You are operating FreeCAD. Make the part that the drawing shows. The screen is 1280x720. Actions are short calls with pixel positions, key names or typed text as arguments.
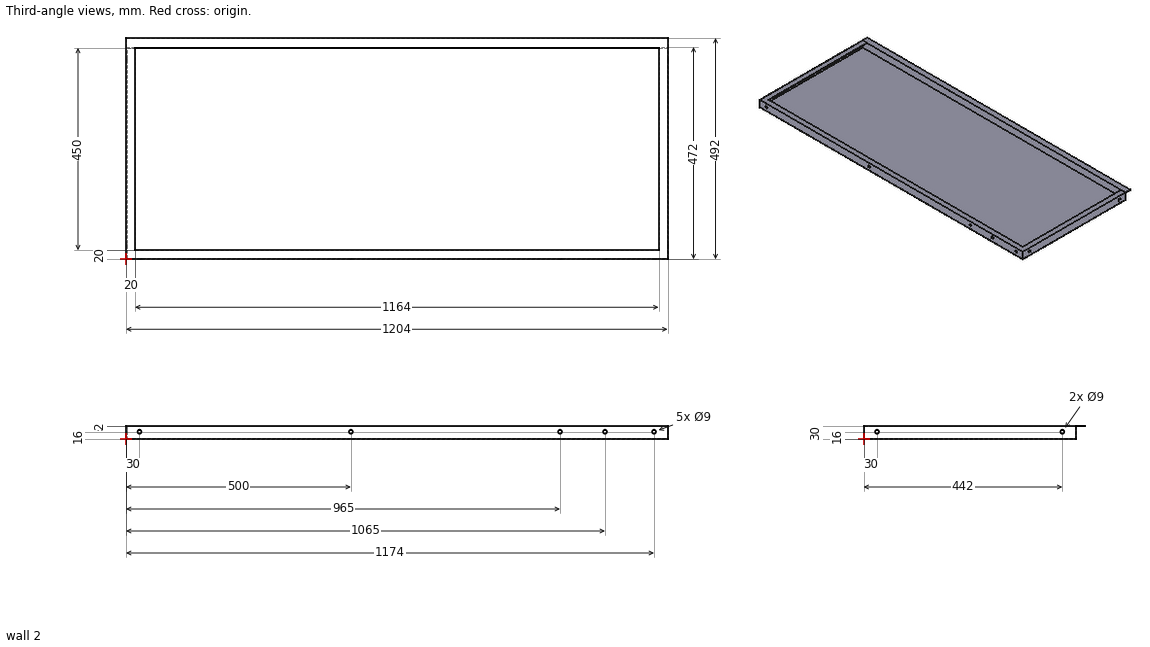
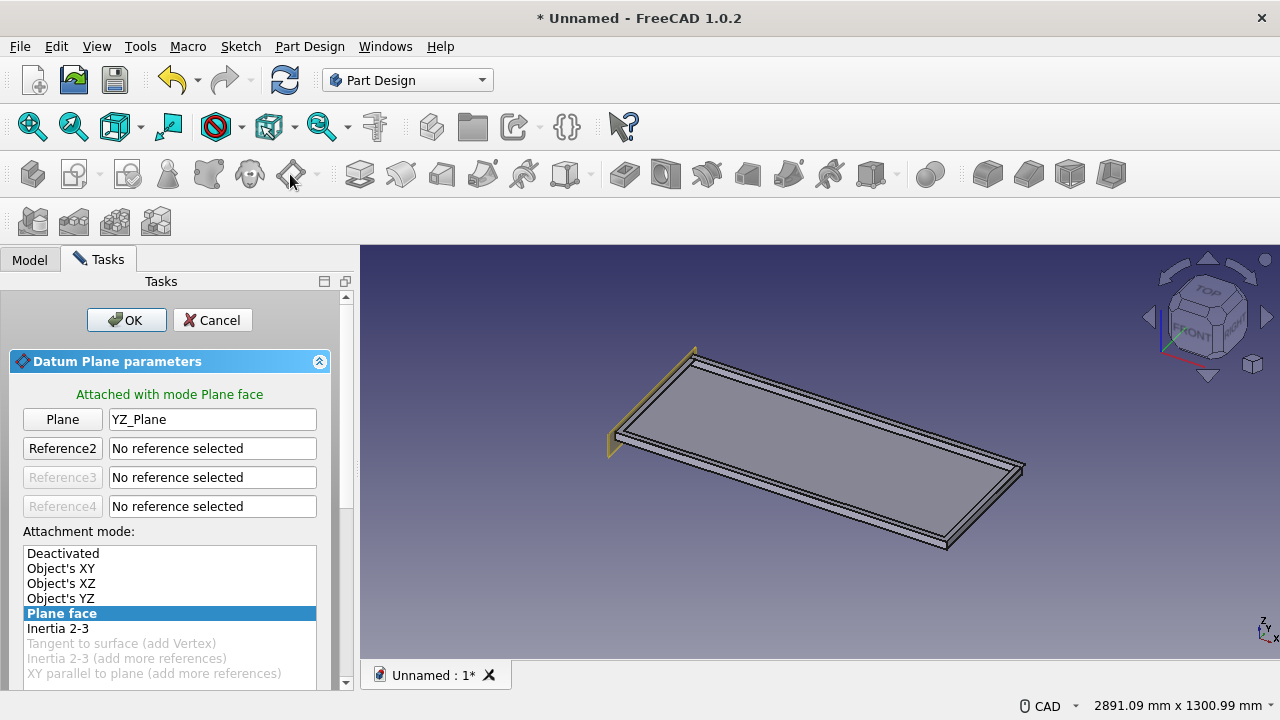
scroll(346, 490, down, 4)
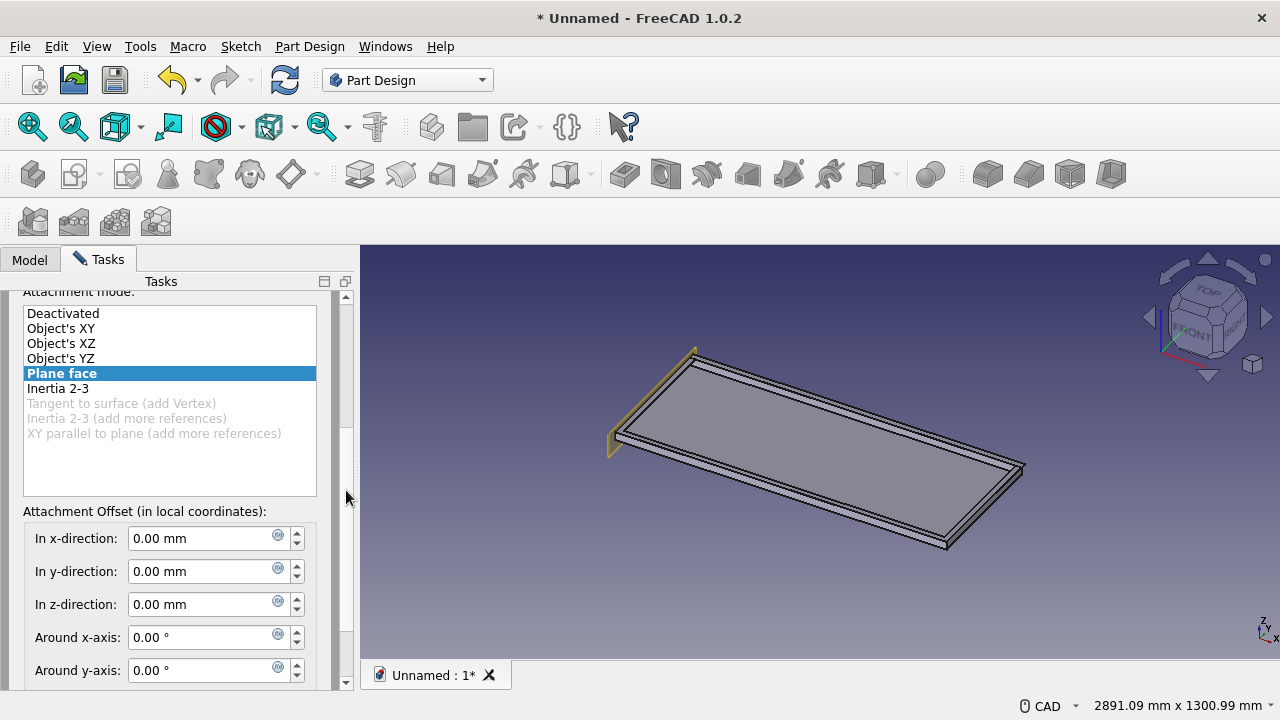
triple_click(210, 604)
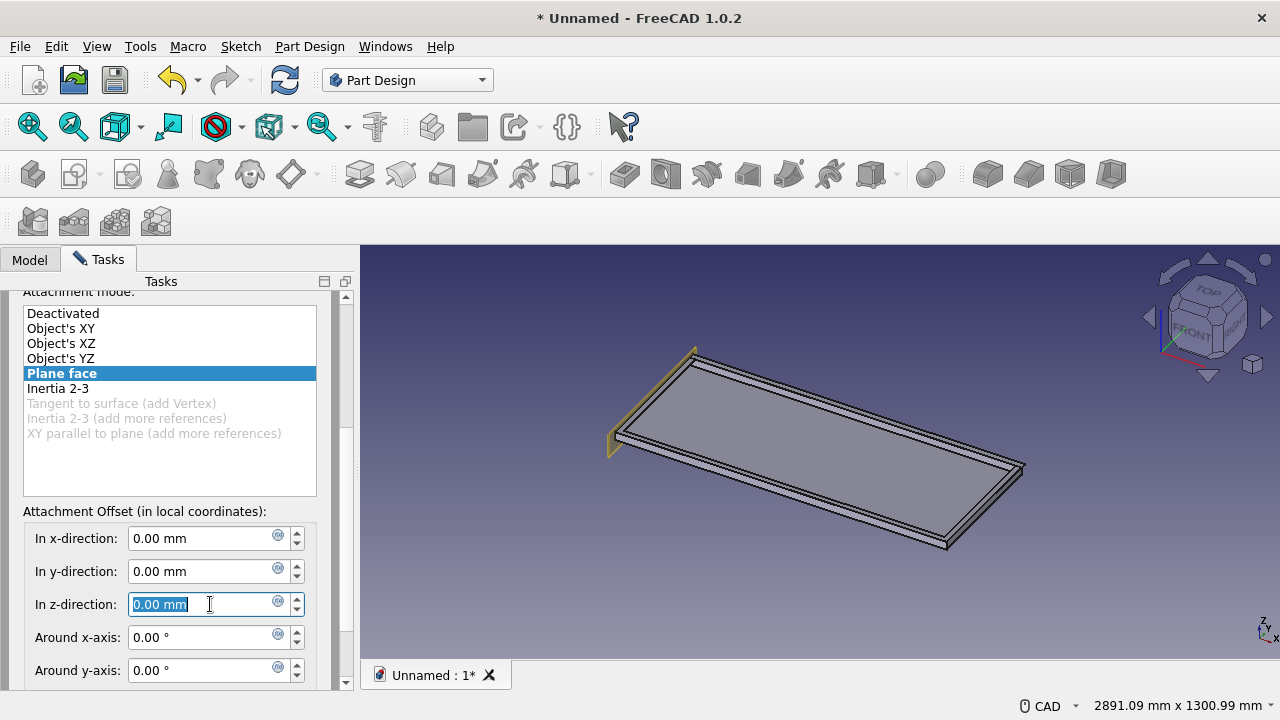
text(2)
key(Tab)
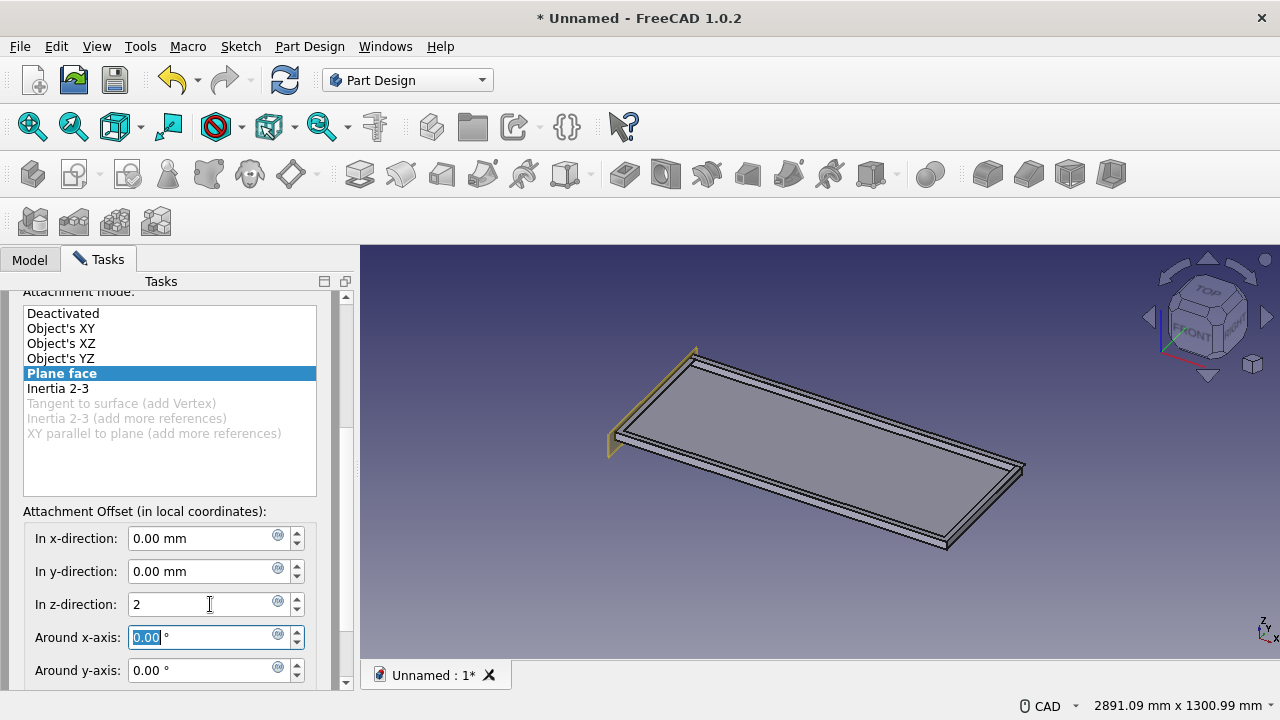
scroll(346, 490, up, 5)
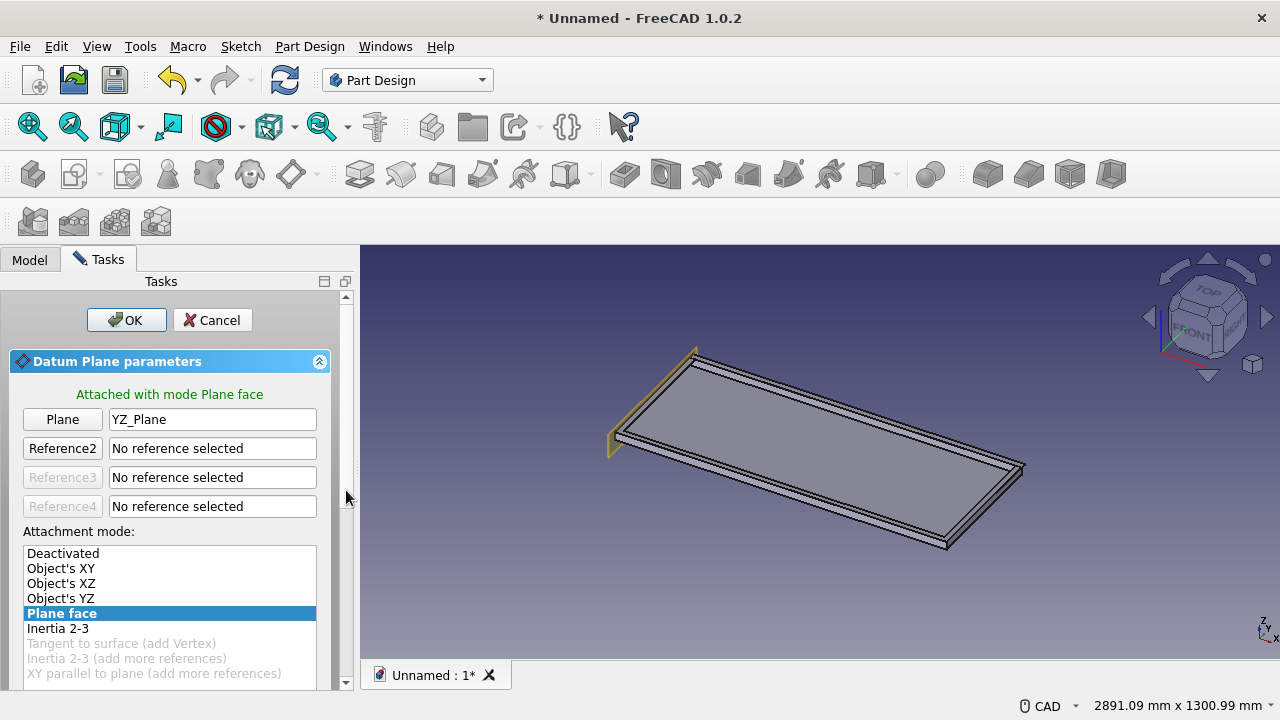
click(127, 320)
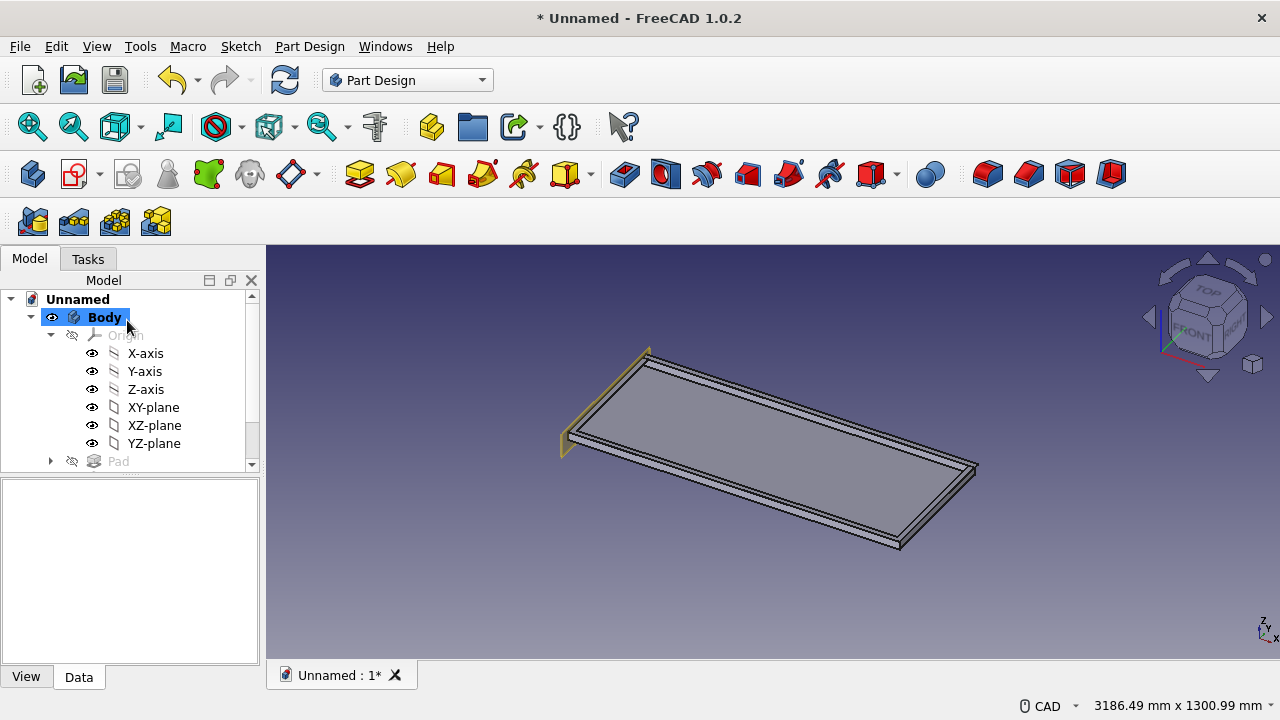
scroll(101, 385, down, 3)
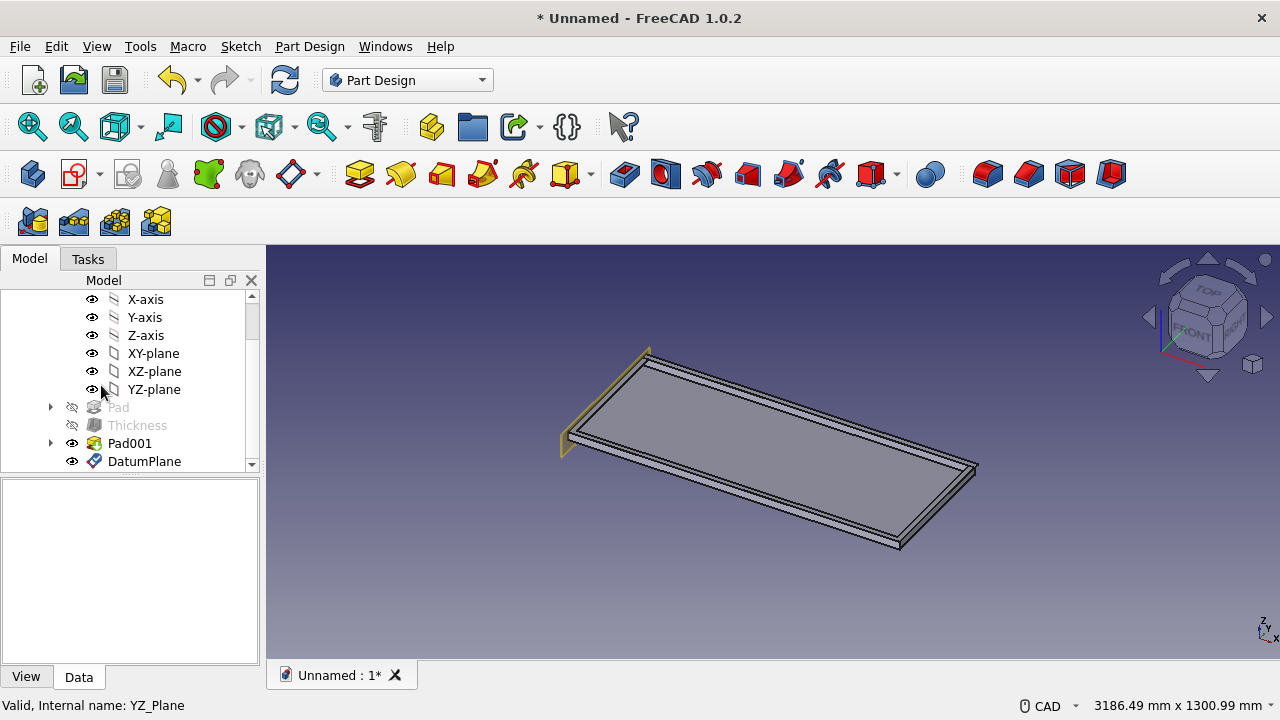
click(117, 461)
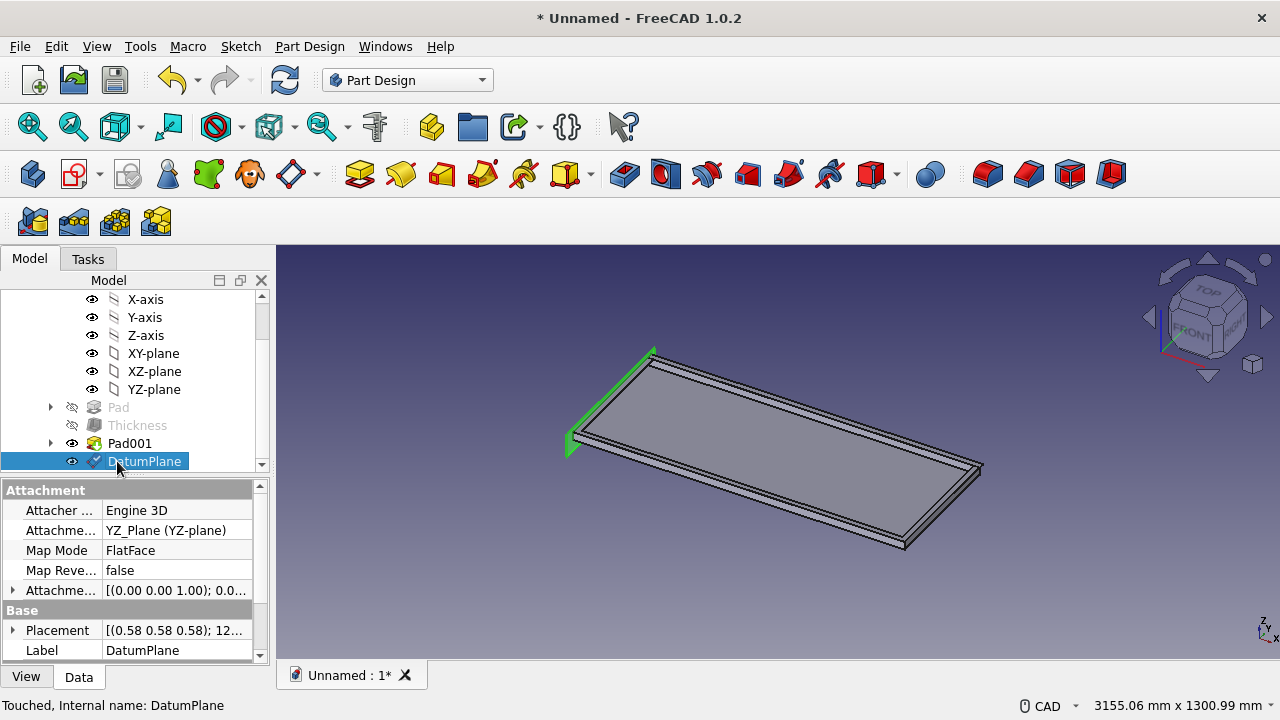
click(74, 174)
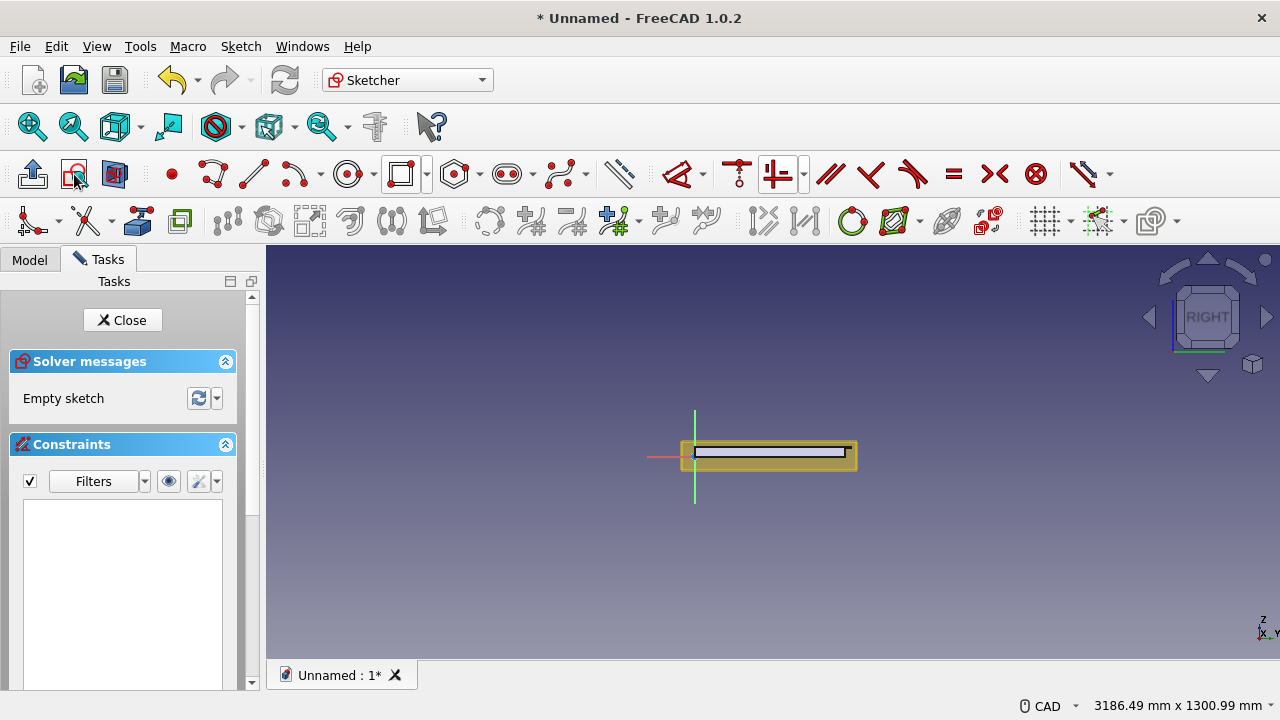
key(q)
key(s)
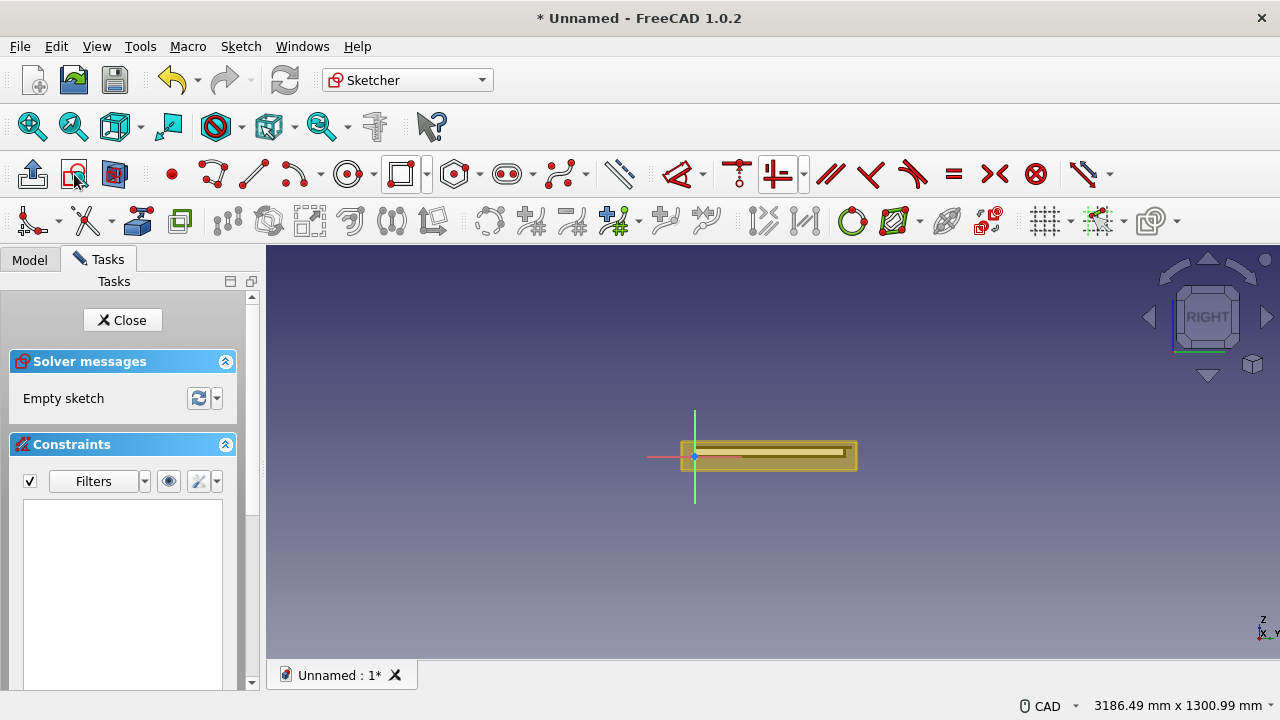
scroll(786, 454, up, 7)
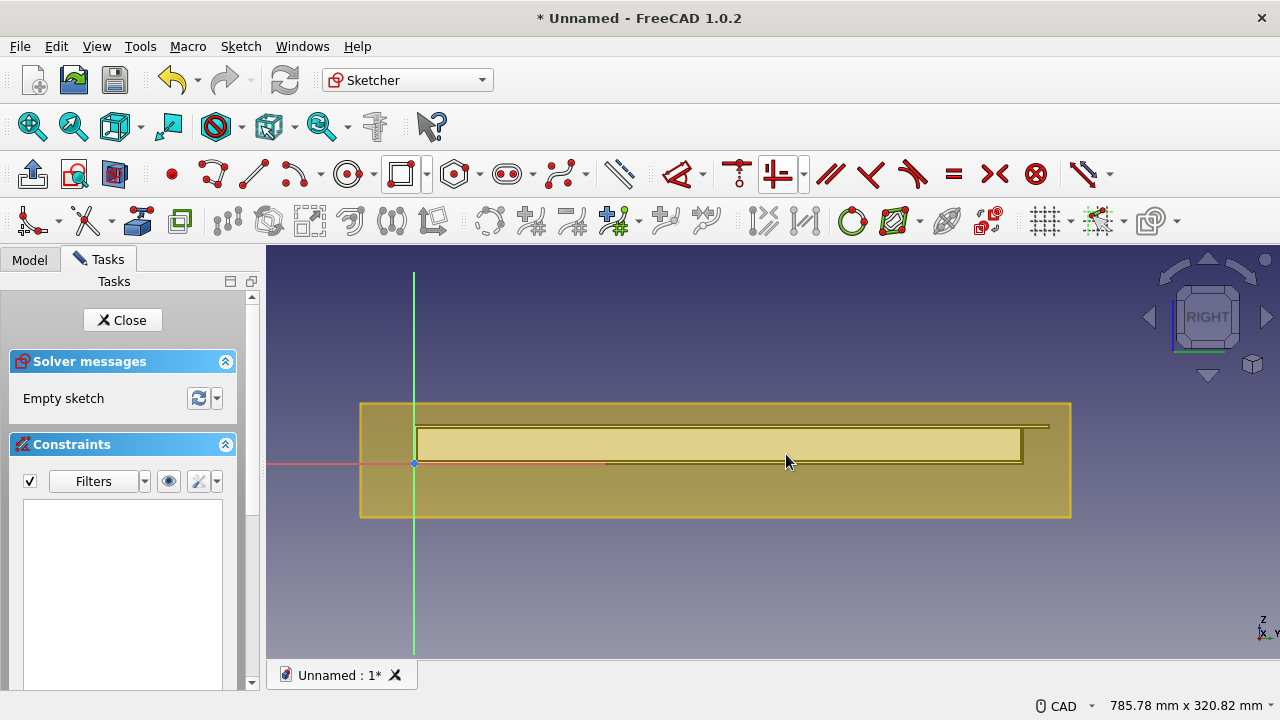
key(g)
key(c)